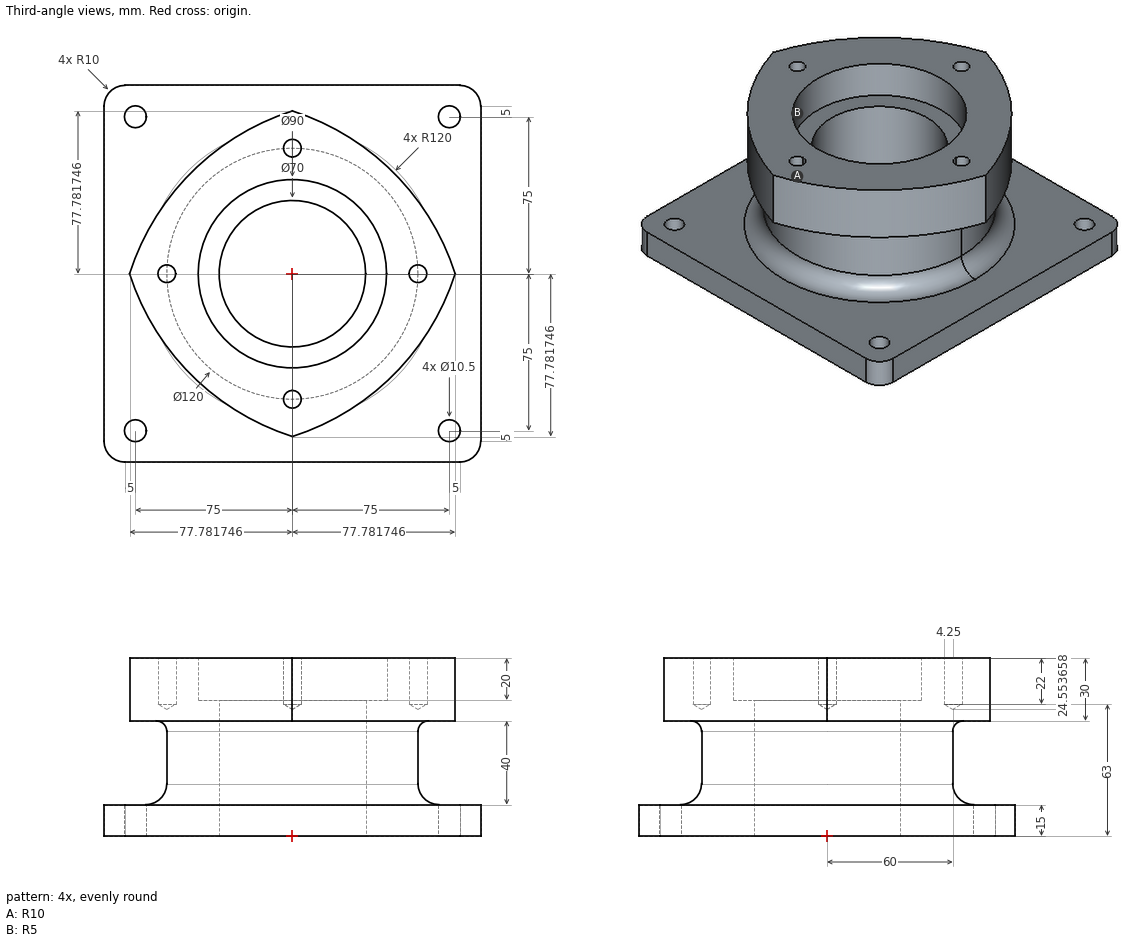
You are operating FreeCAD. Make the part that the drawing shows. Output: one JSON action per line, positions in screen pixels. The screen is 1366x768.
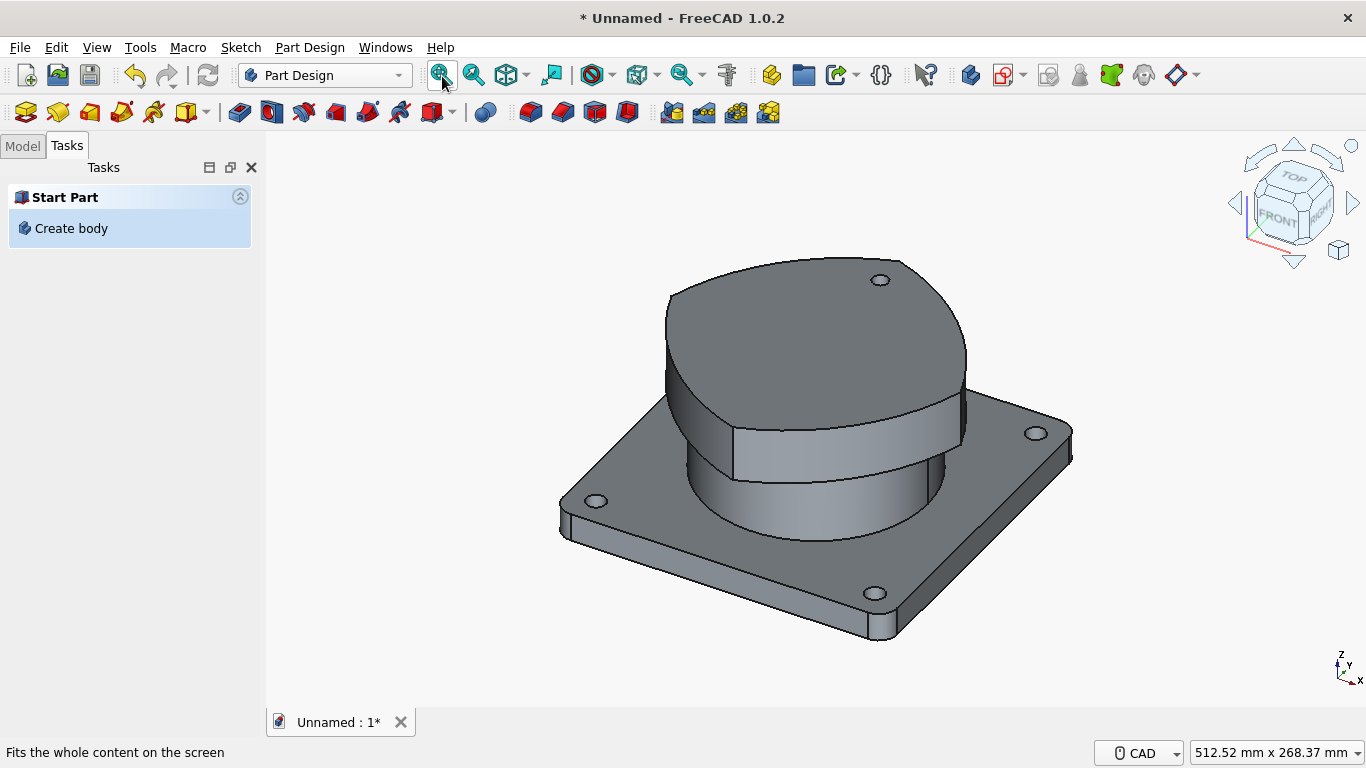
{"action": "left_click", "coordinate": [23, 145]}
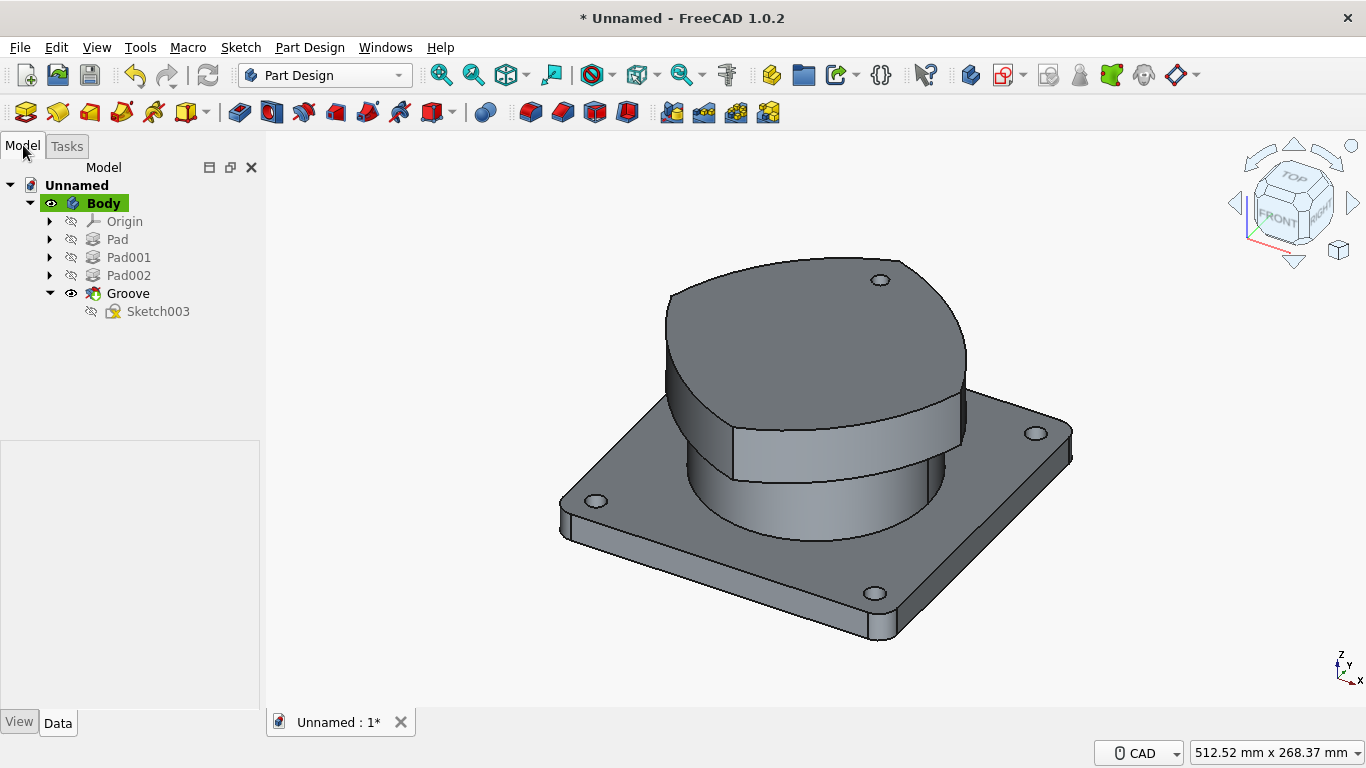
{"action": "left_click", "coordinate": [116, 293]}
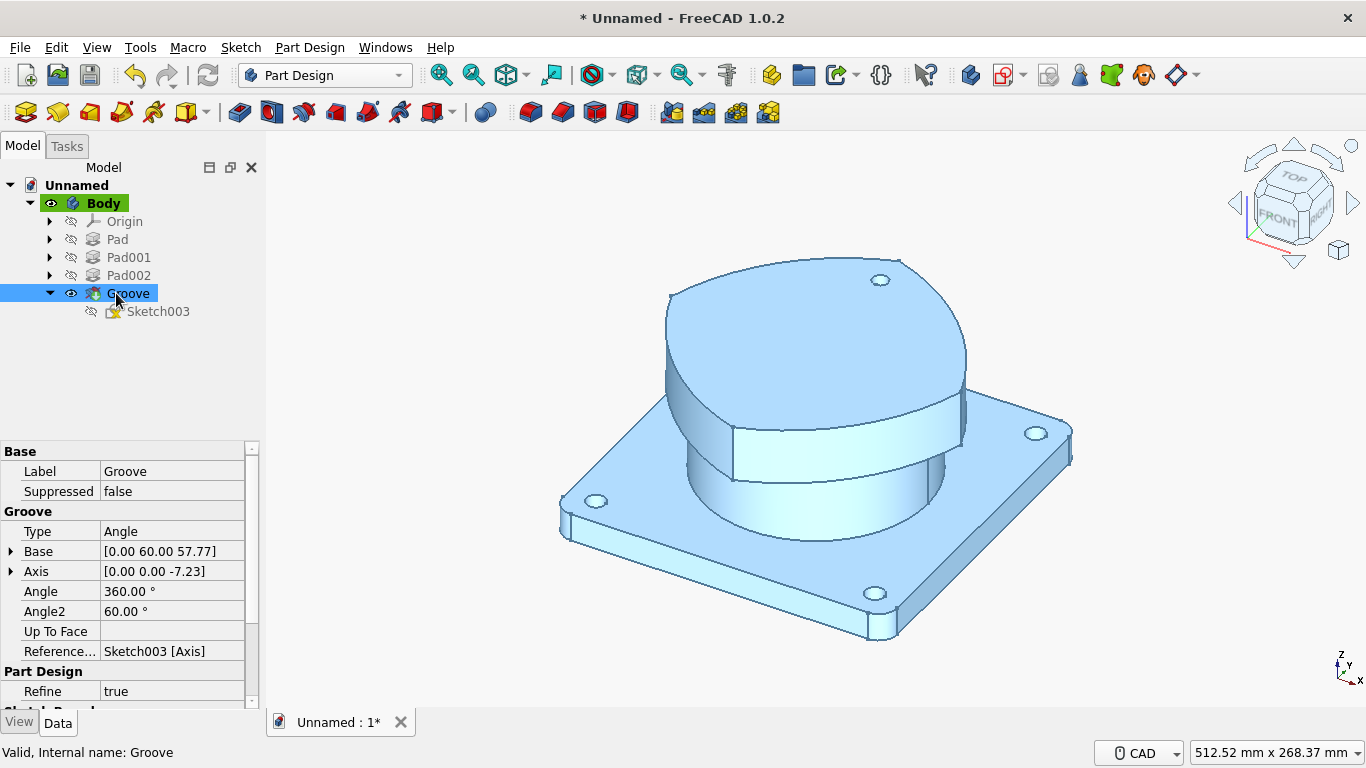
{"action": "left_click", "coordinate": [736, 112]}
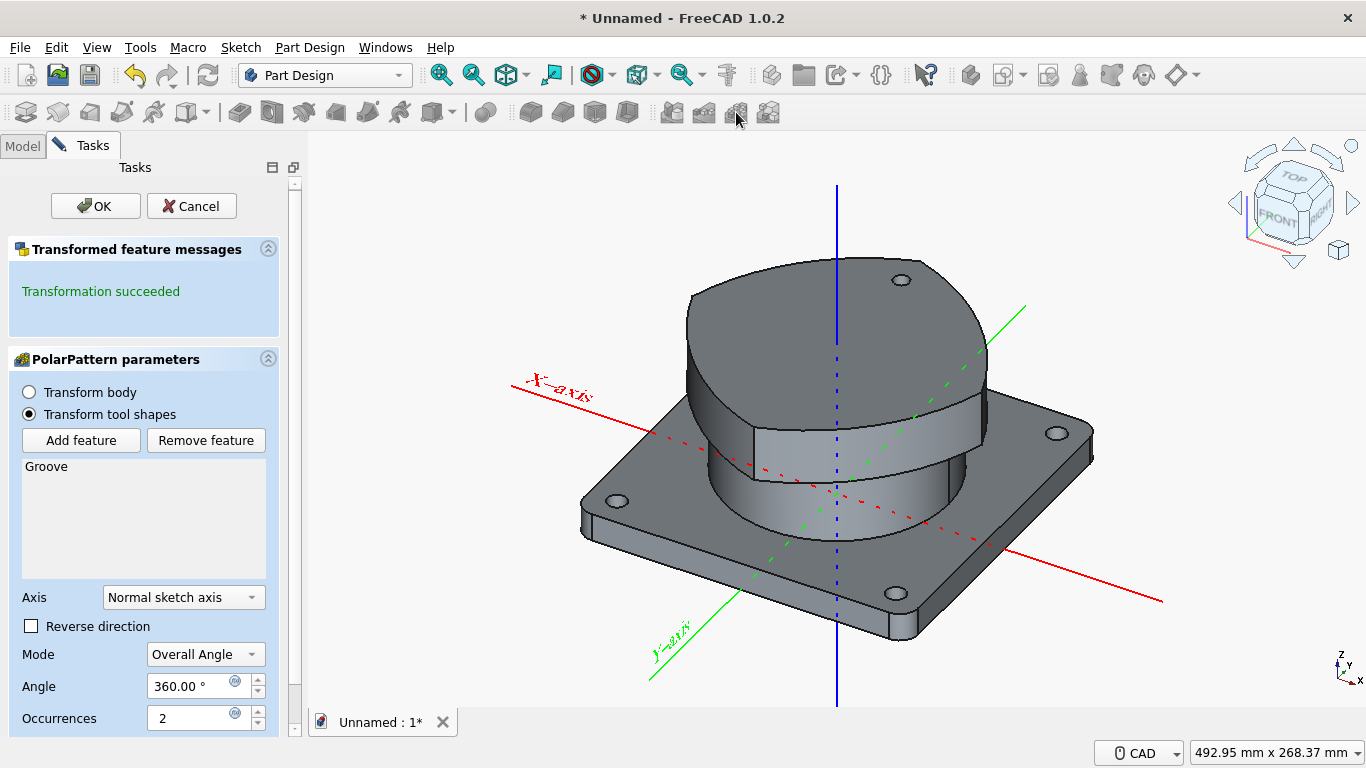
{"action": "left_click", "coordinate": [184, 598]}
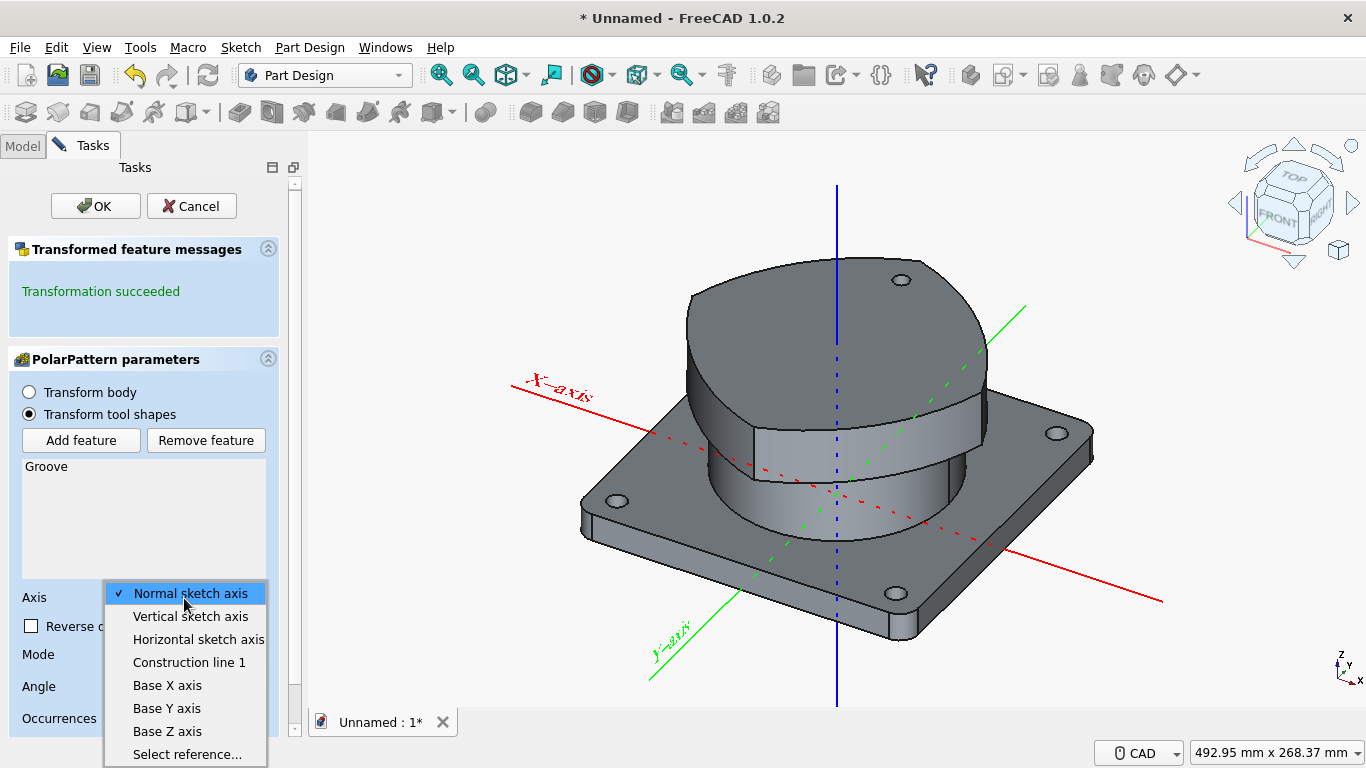
{"action": "left_click", "coordinate": [184, 732]}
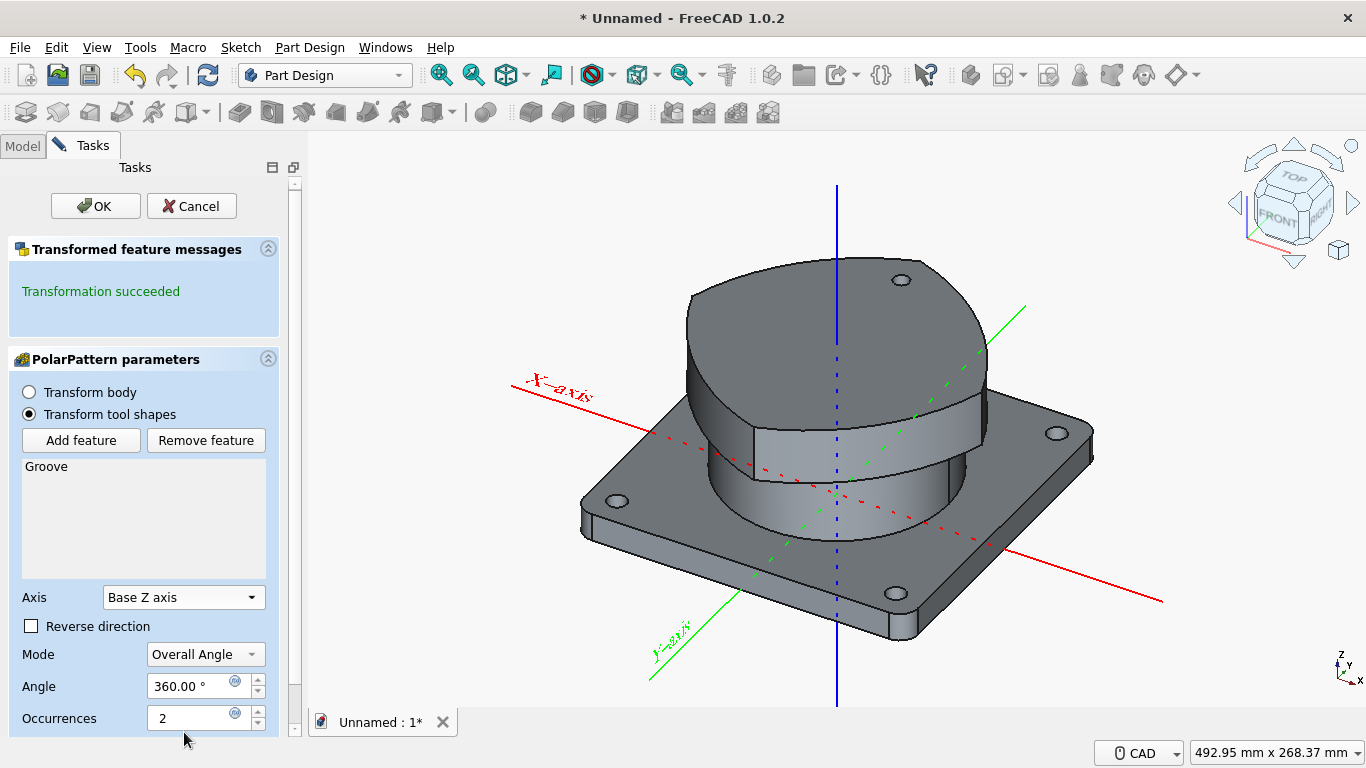
{"action": "triple_click", "coordinate": [198, 718]}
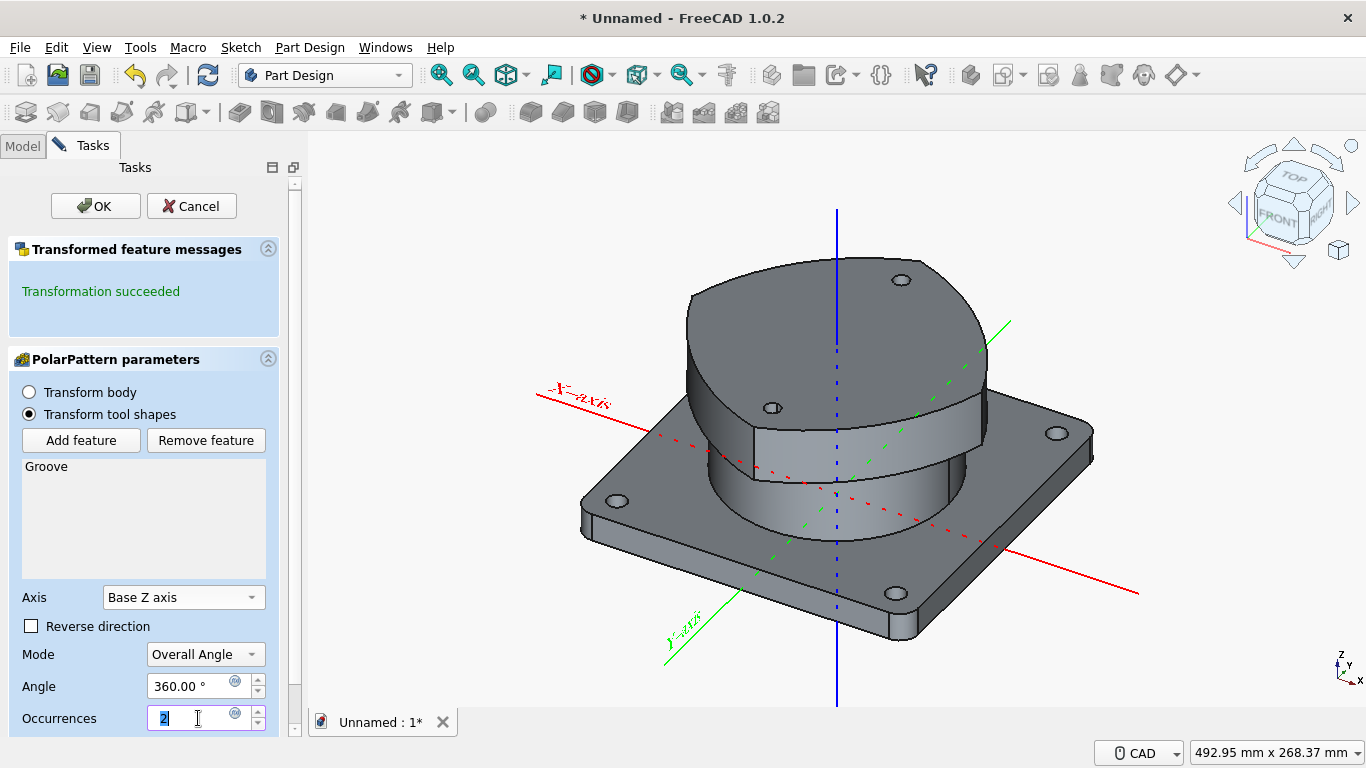
{"action": "type", "text": "4"}
{"action": "key", "text": "Tab"}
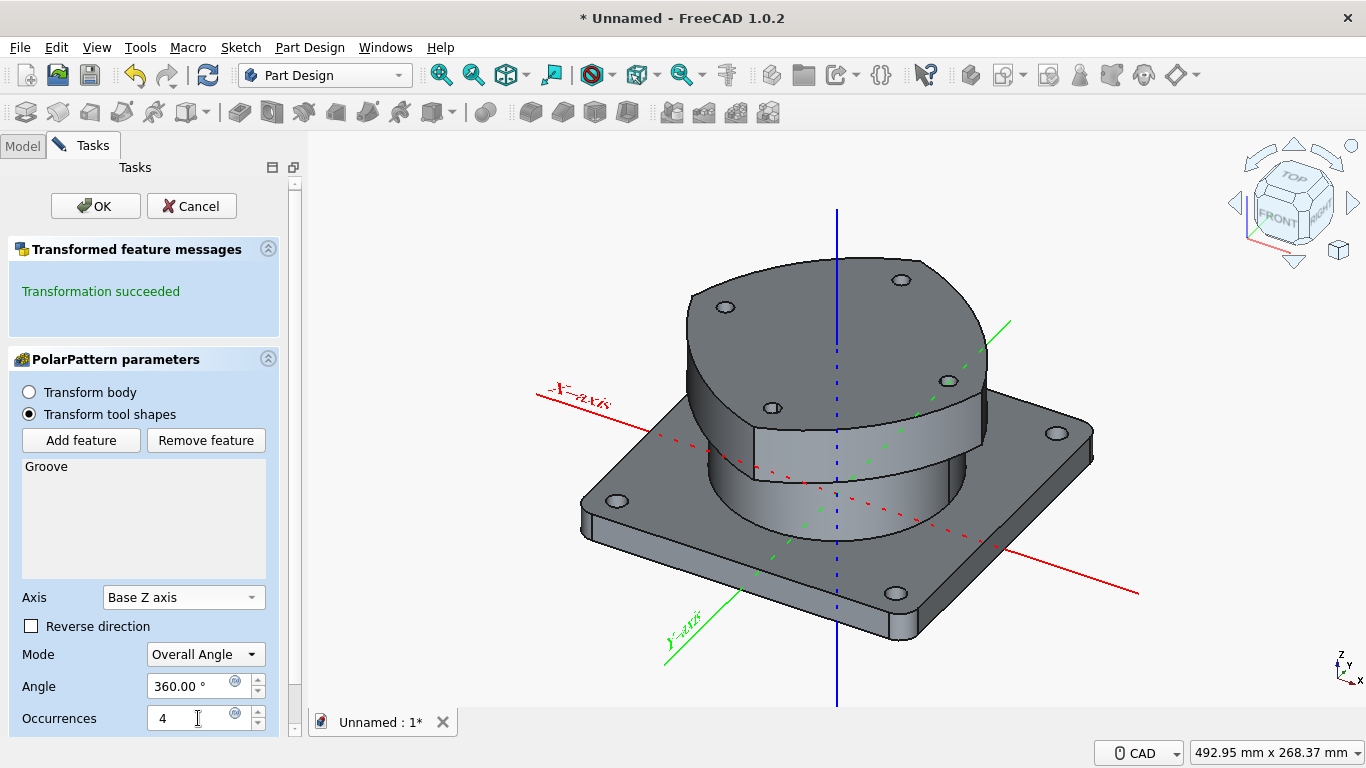
{"action": "left_click", "coordinate": [96, 206]}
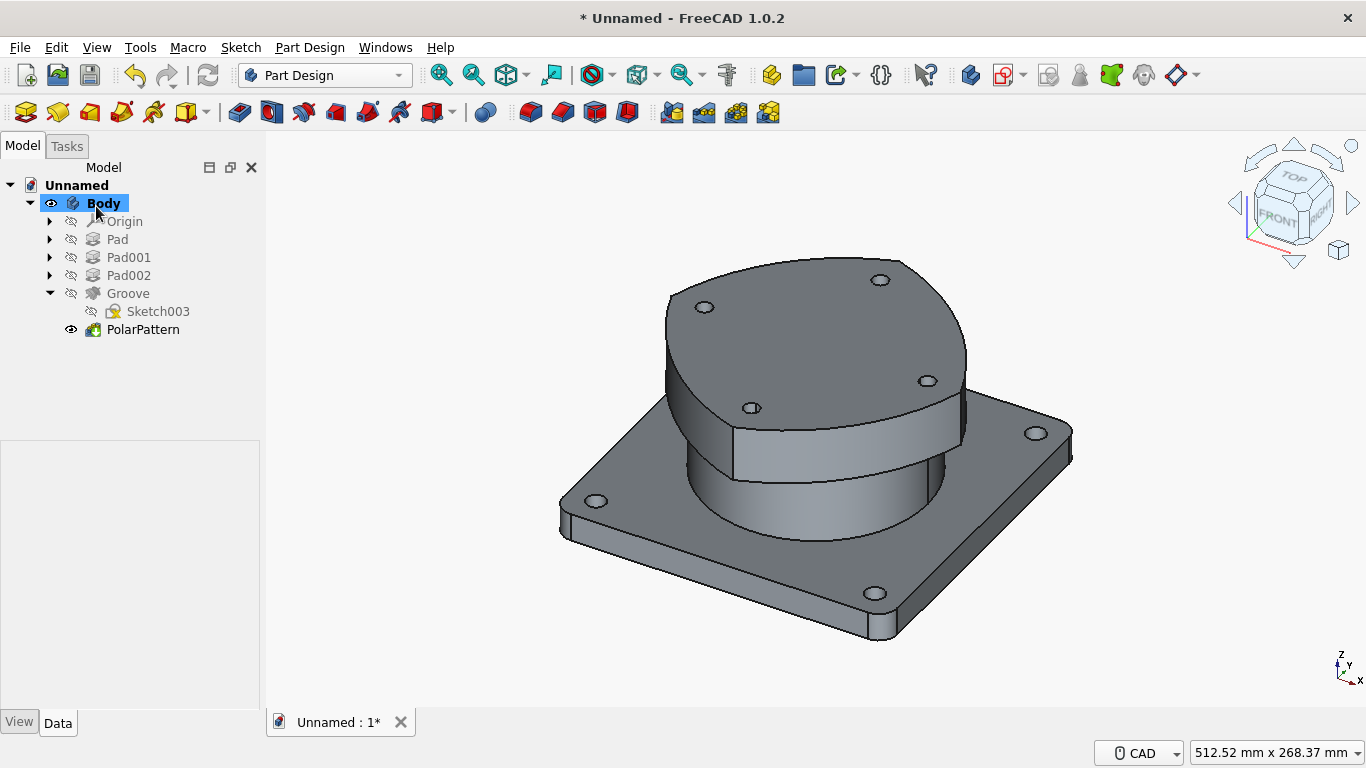
{"action": "key", "text": "0"}